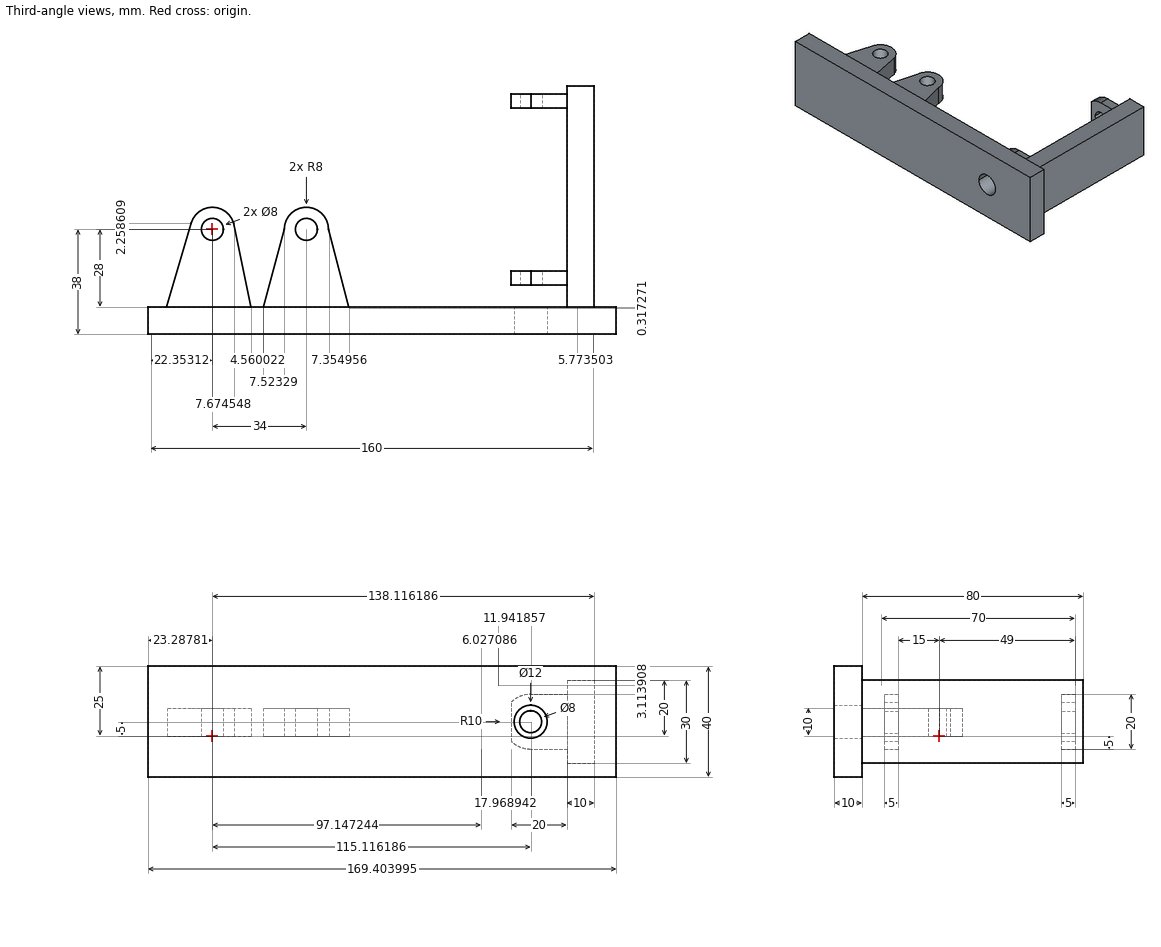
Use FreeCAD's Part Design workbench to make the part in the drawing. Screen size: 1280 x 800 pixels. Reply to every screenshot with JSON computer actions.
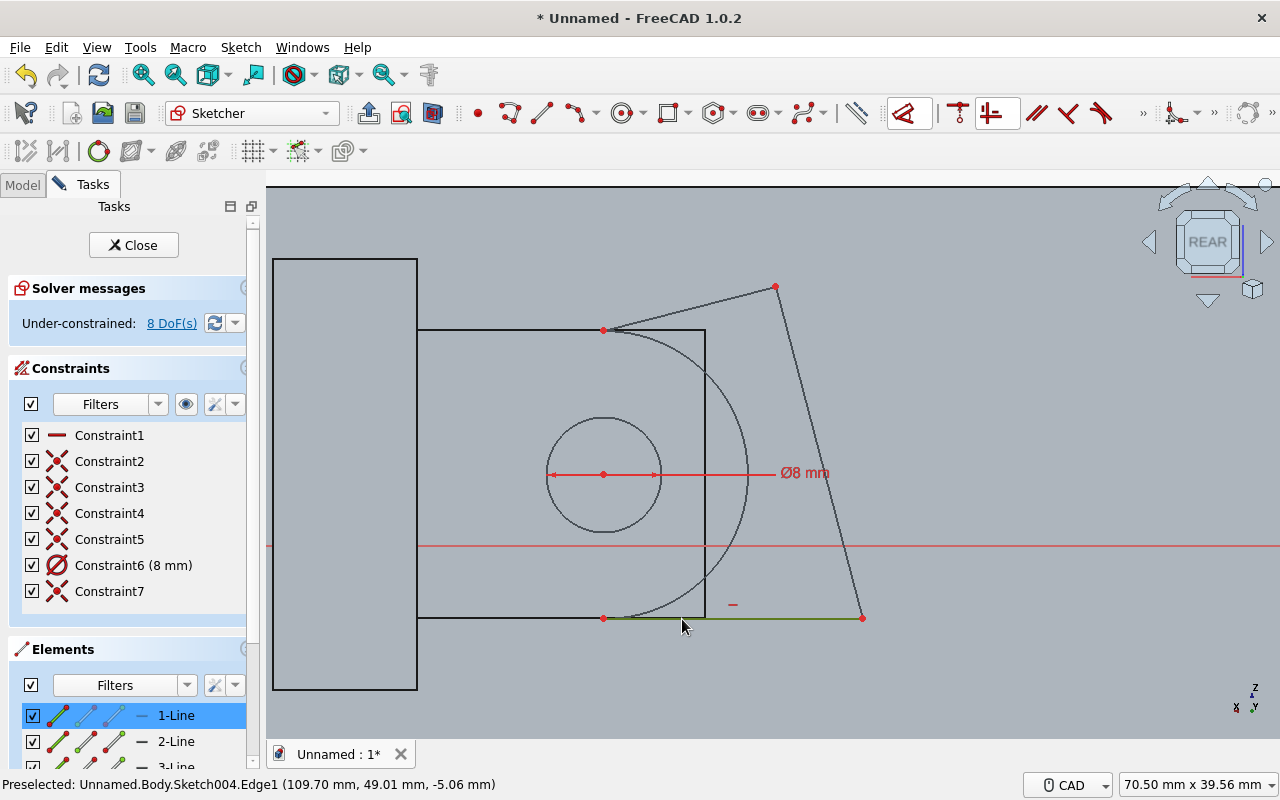
{"action": "left_click", "coordinate": [720, 560]}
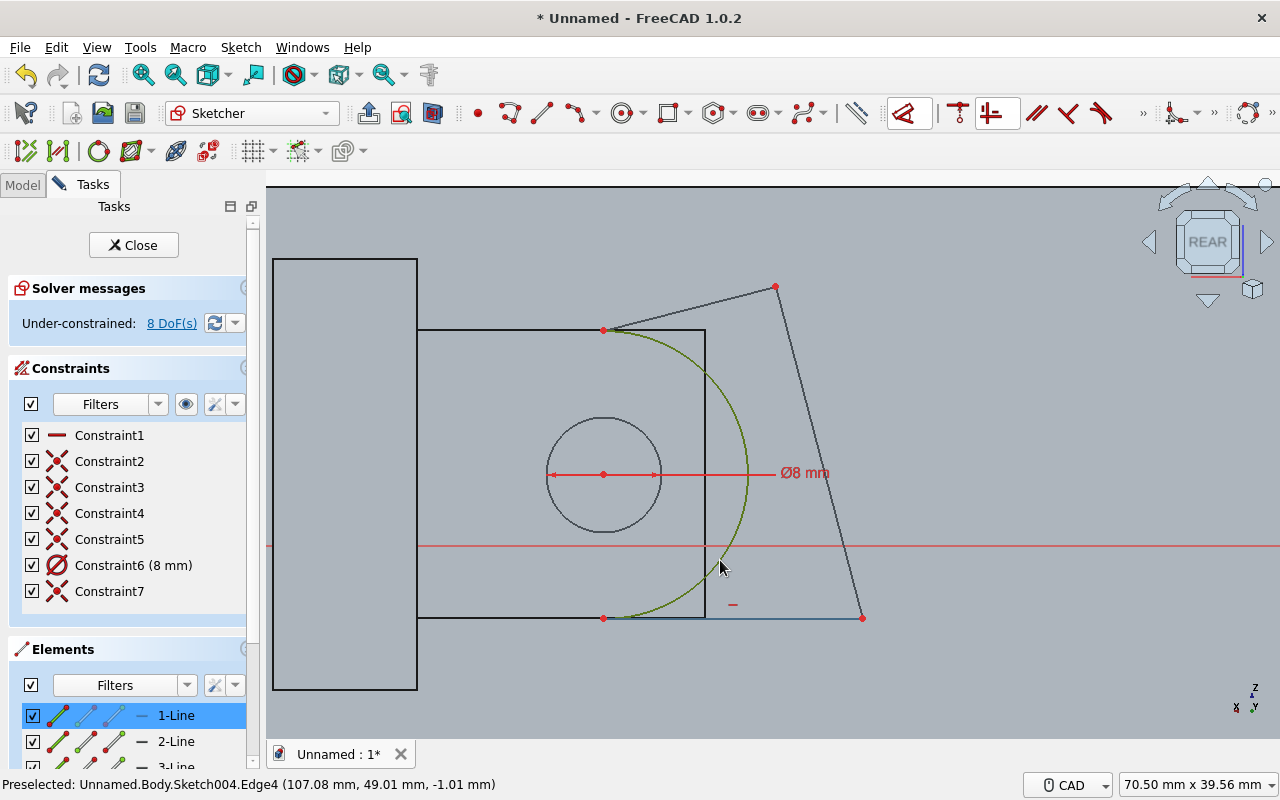
{"action": "left_click", "coordinate": [1102, 114]}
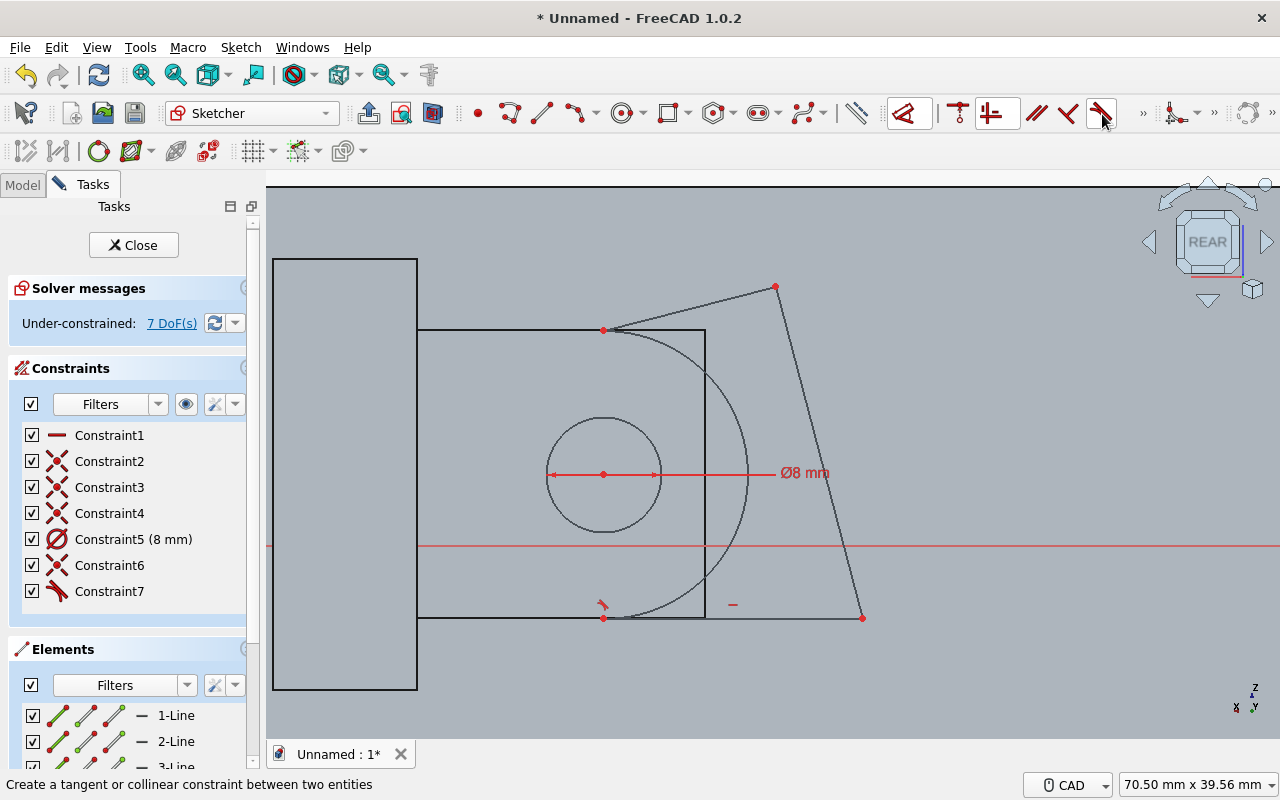
{"action": "left_click", "coordinate": [720, 560]}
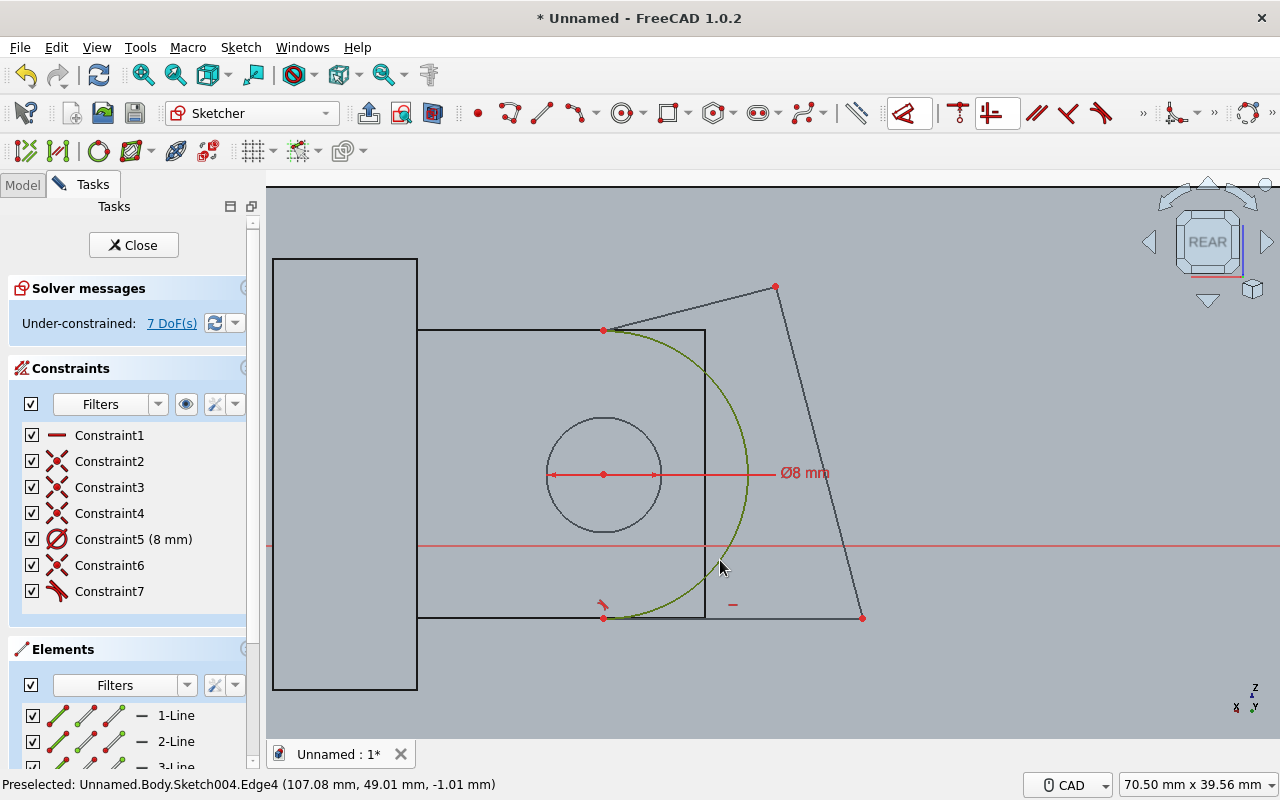
{"action": "left_click", "coordinate": [926, 114]}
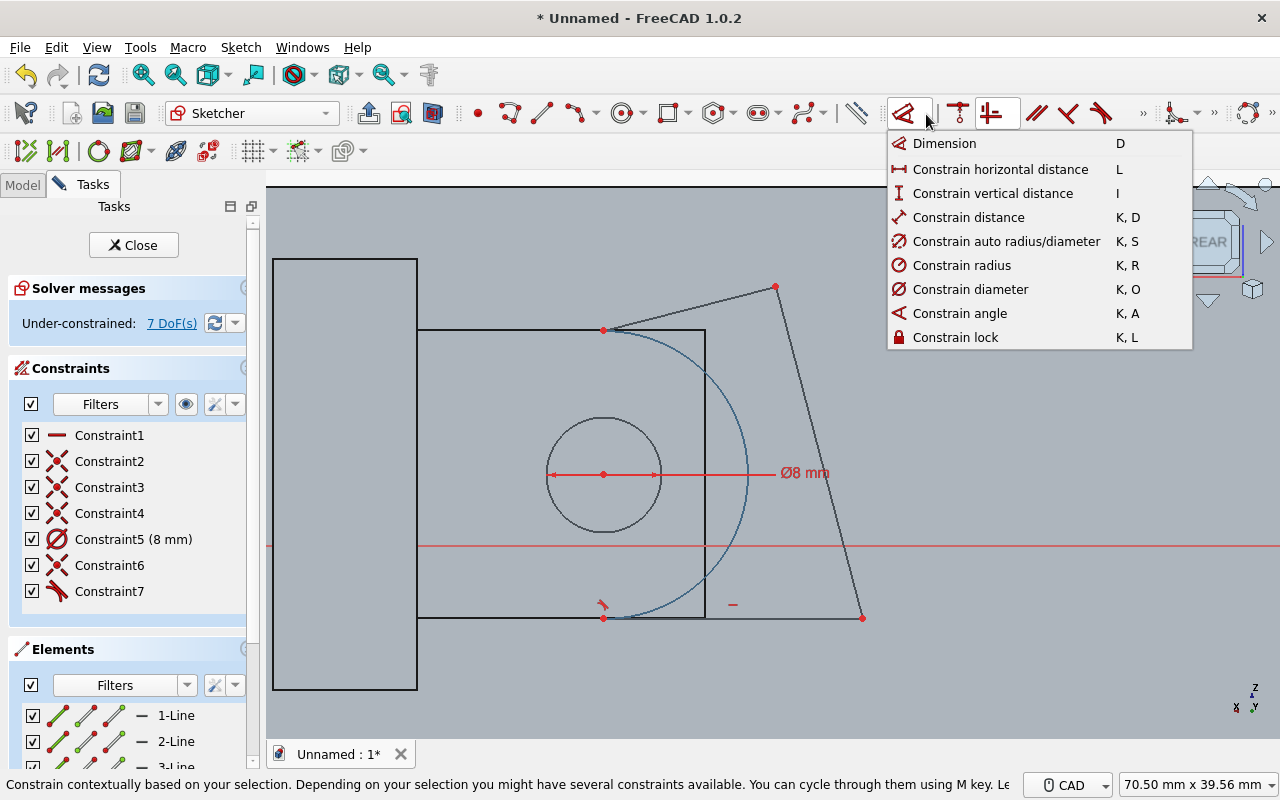
{"action": "left_click", "coordinate": [1040, 265]}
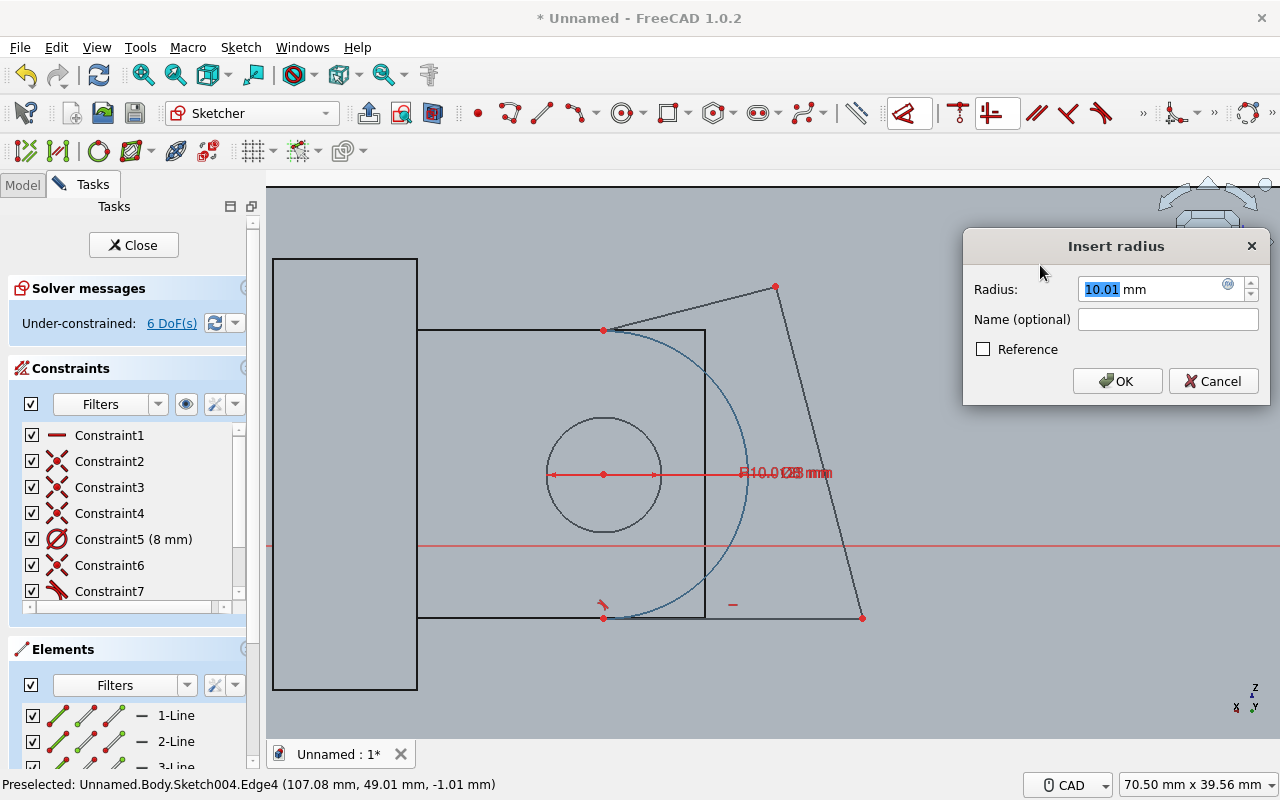
{"action": "type", "text": "10"}
{"action": "key", "text": "Return"}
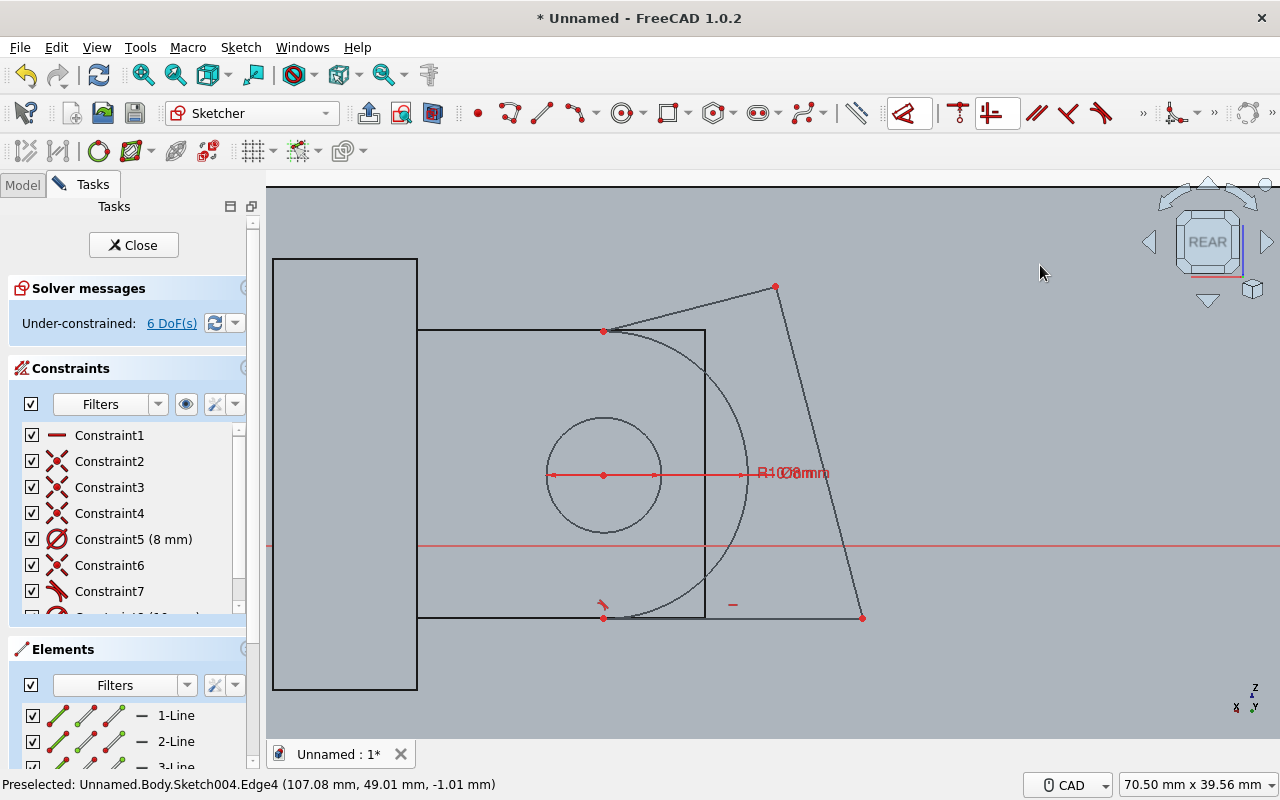
{"action": "left_click", "coordinate": [604, 475]}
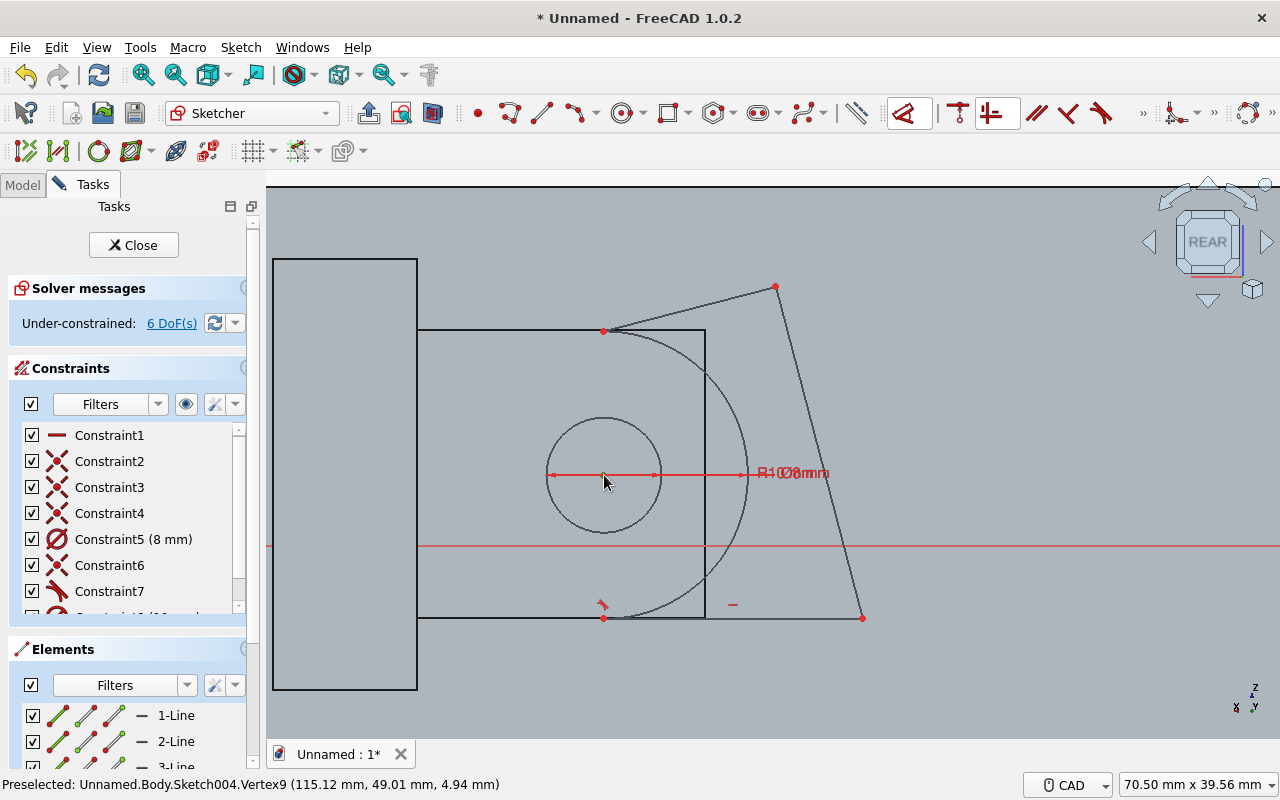
{"action": "left_click", "coordinate": [926, 114]}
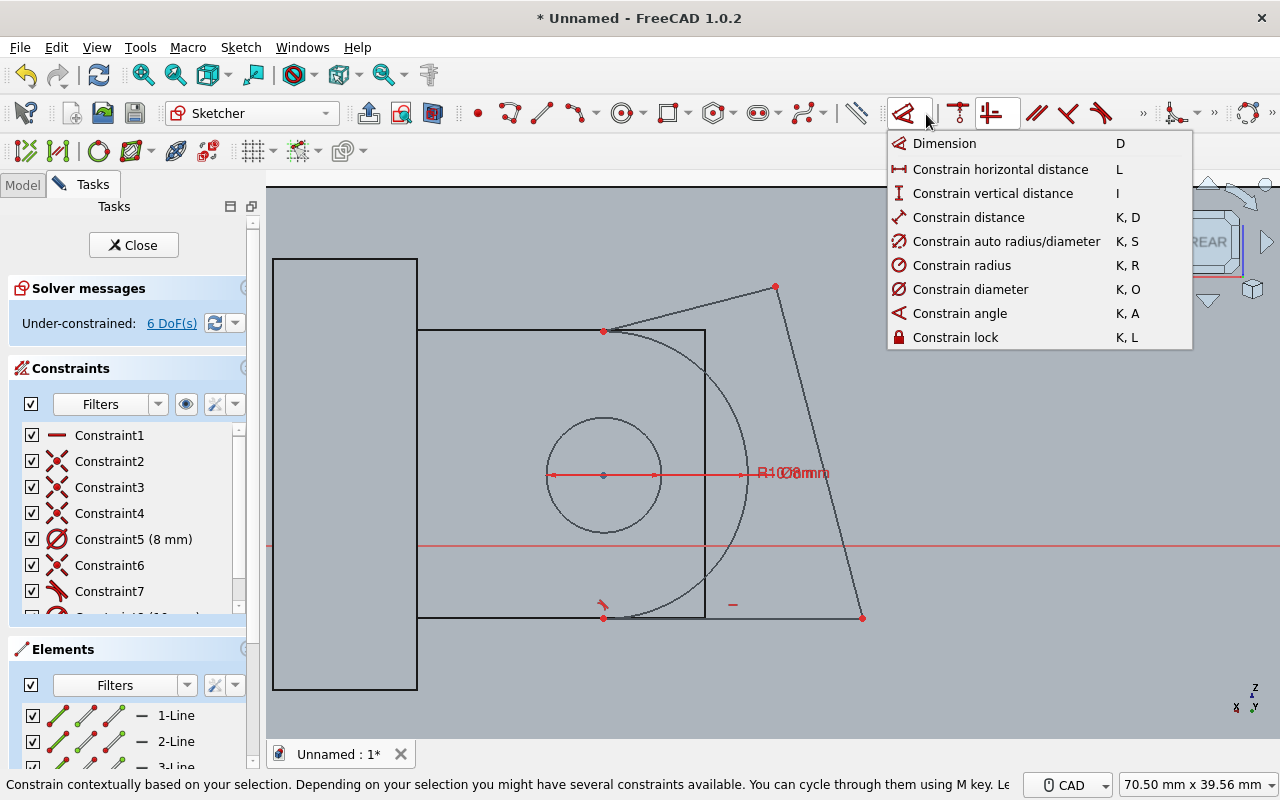
{"action": "left_click", "coordinate": [1040, 193]}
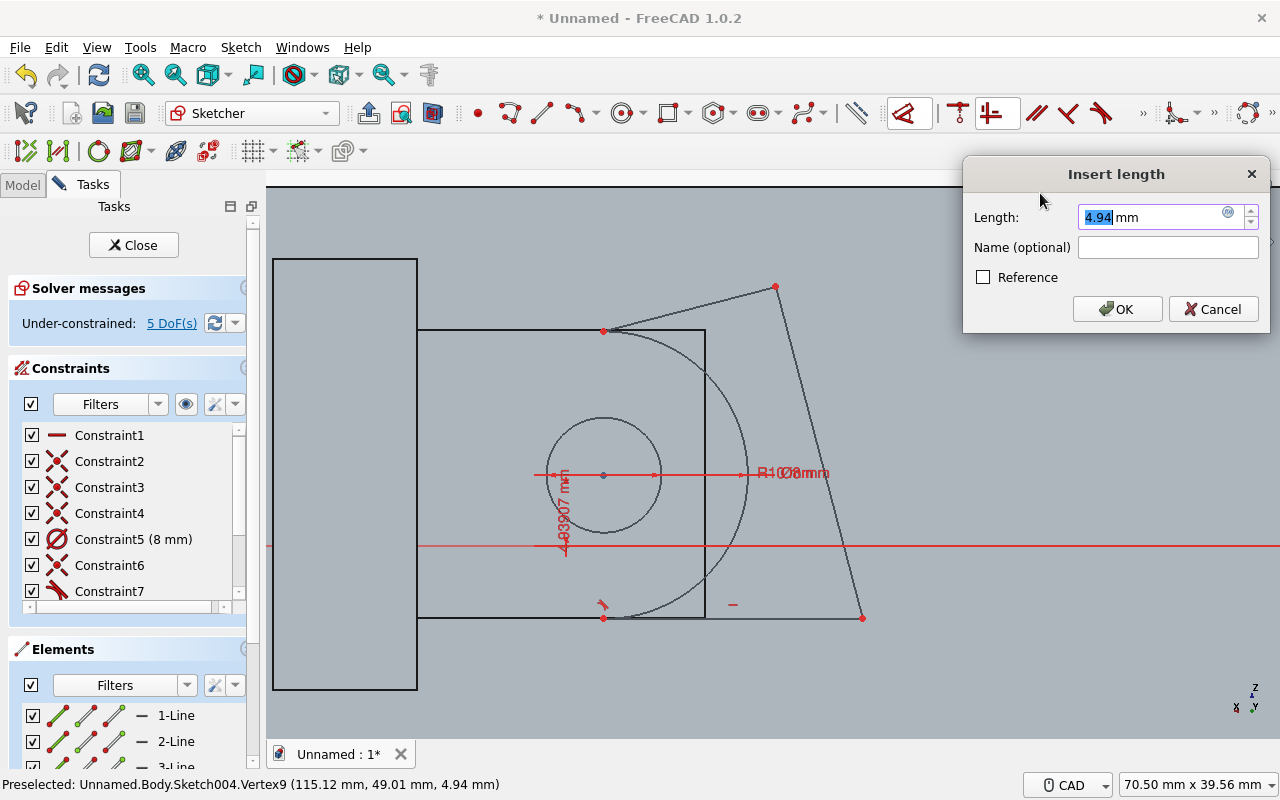
{"action": "type", "text": "5"}
{"action": "key", "text": "Return"}